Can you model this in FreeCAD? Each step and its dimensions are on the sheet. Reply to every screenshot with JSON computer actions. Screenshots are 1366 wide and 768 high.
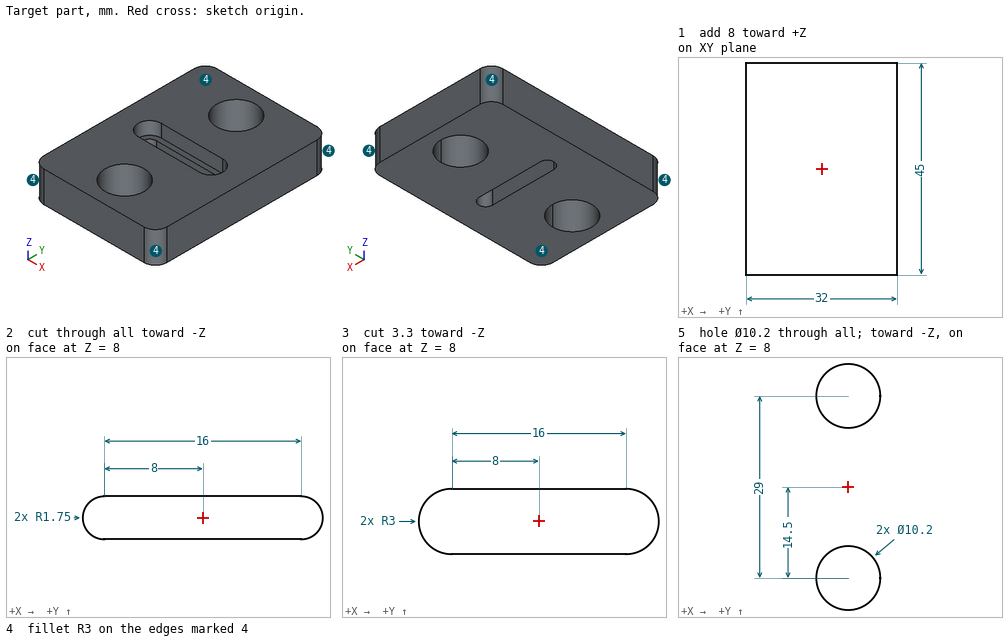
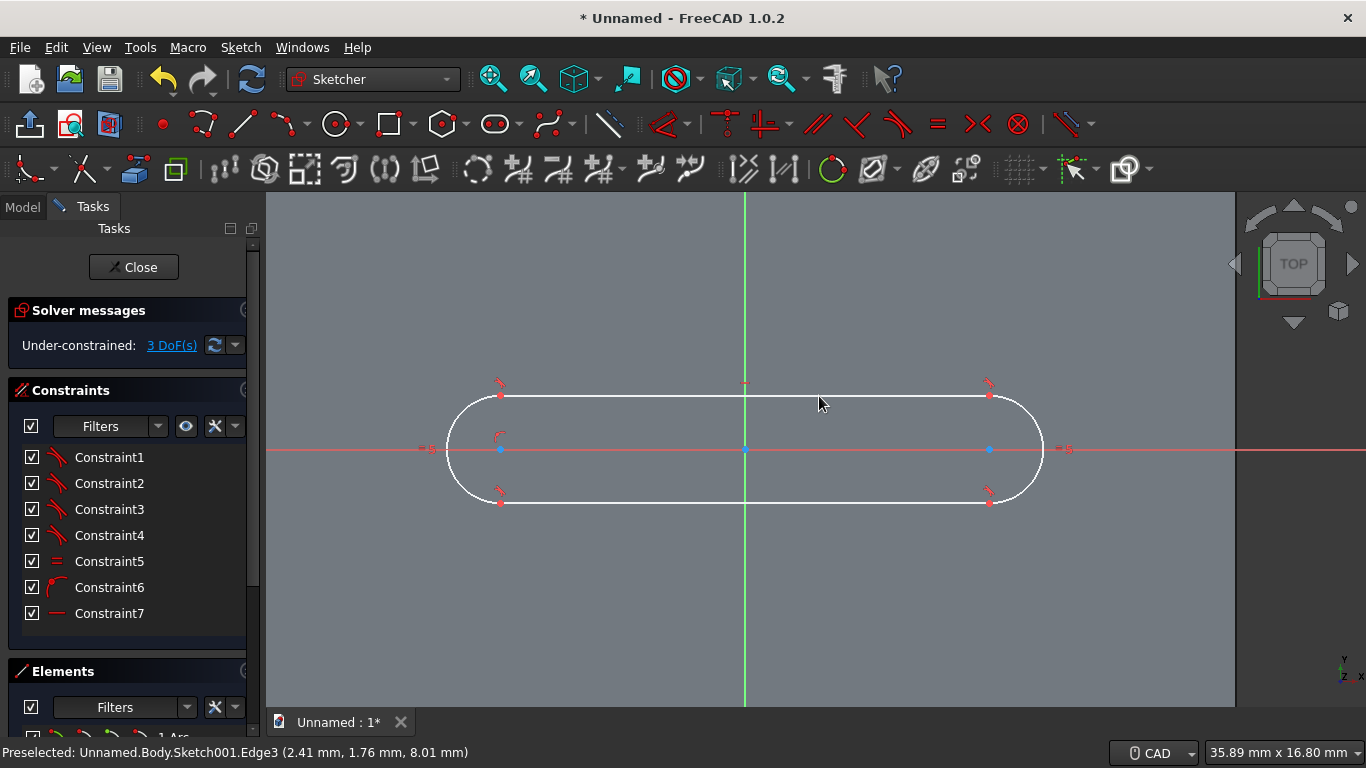
{"action": "key", "text": "d"}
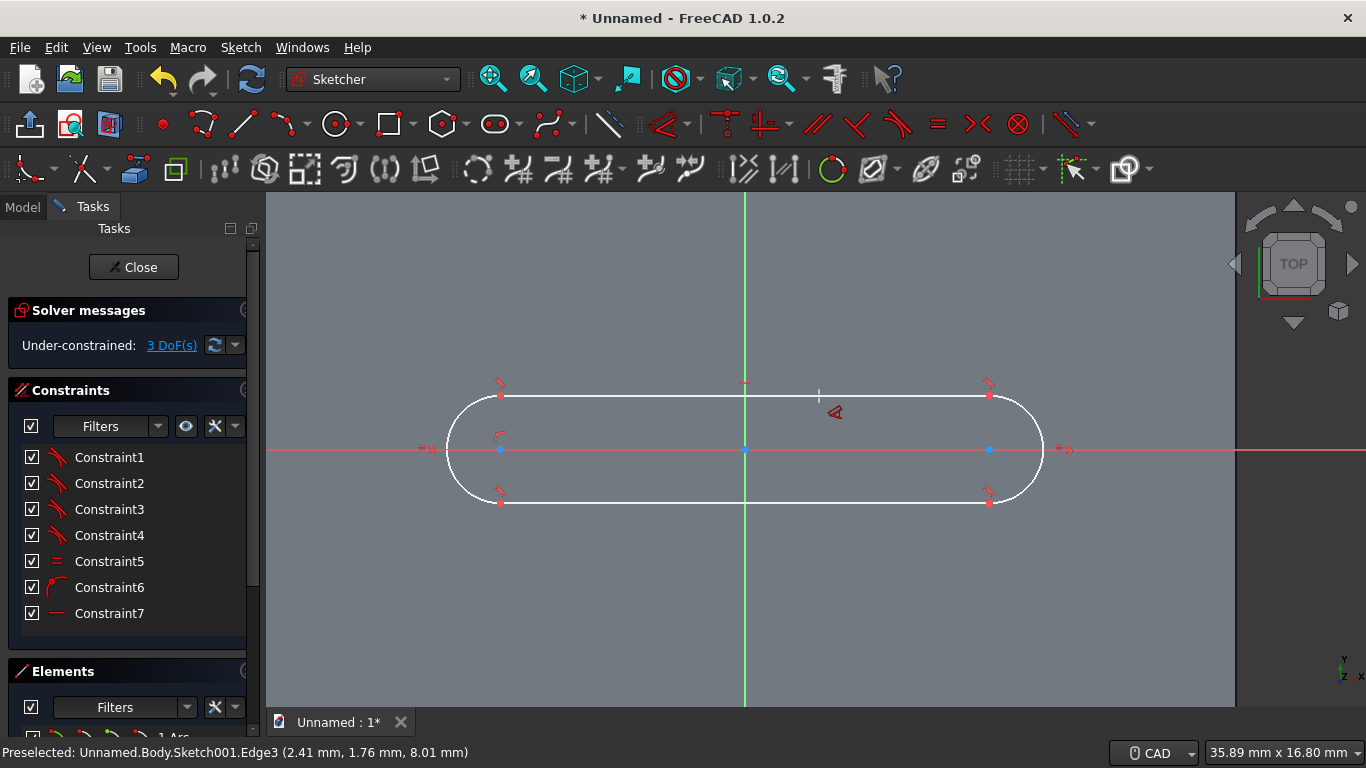
{"action": "left_click", "coordinate": [457, 418]}
{"action": "left_click", "coordinate": [431, 399]}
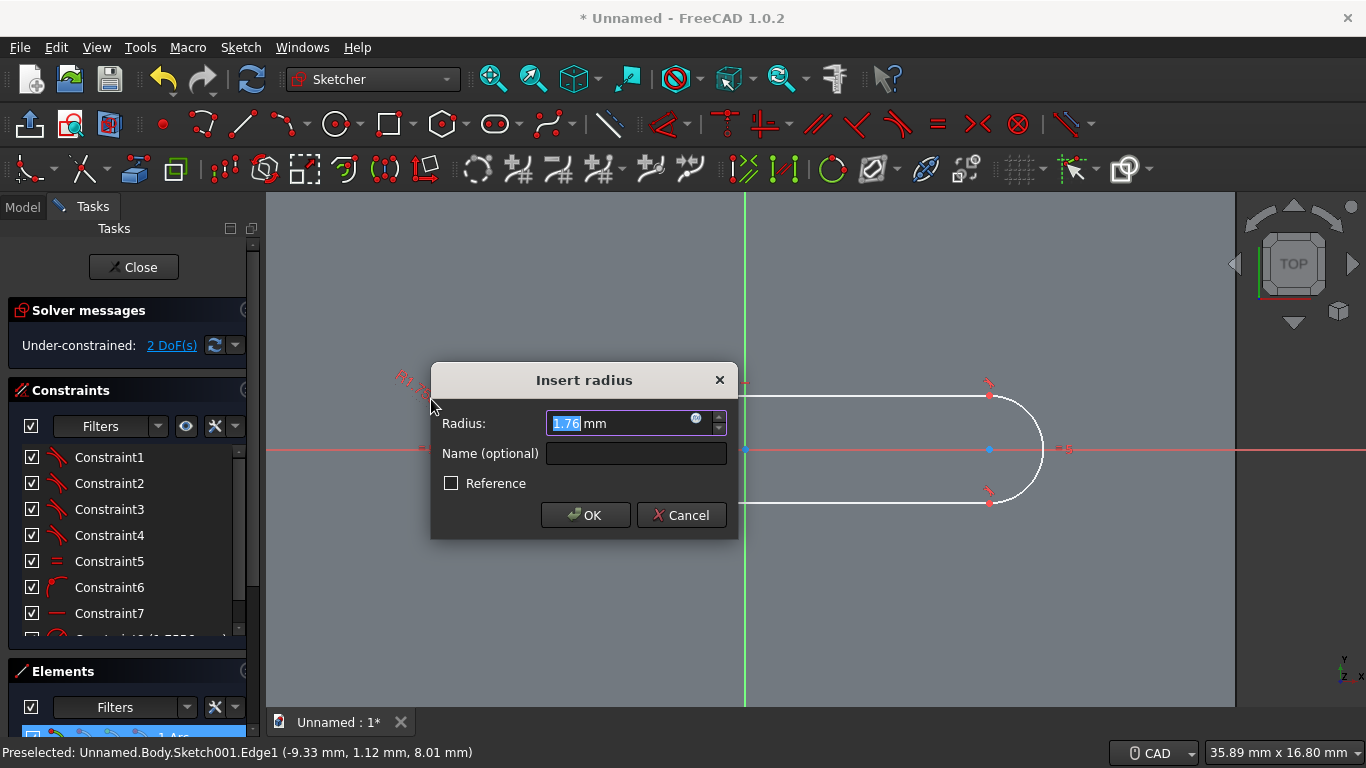
{"action": "type", "text": "1.75"}
{"action": "key", "text": "Return"}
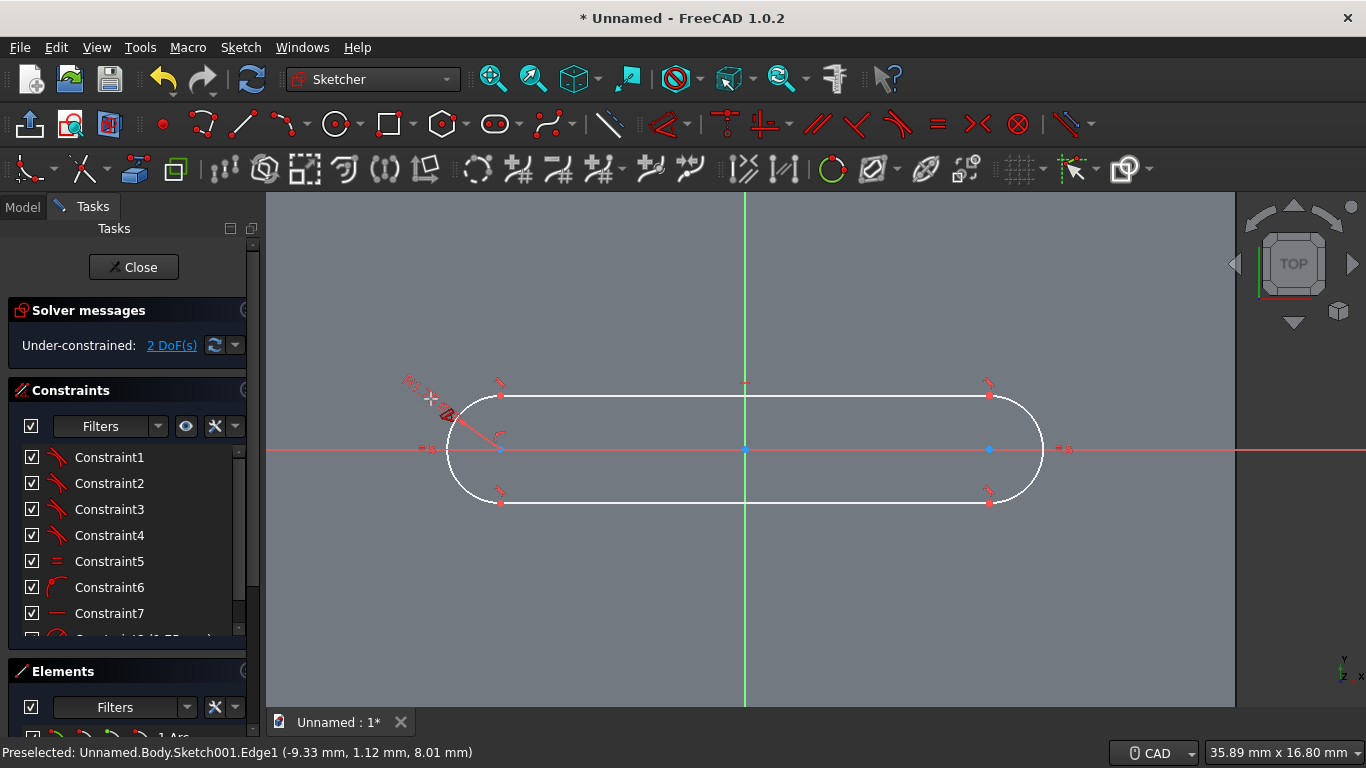
{"action": "left_click", "coordinate": [647, 396]}
{"action": "left_click", "coordinate": [633, 362]}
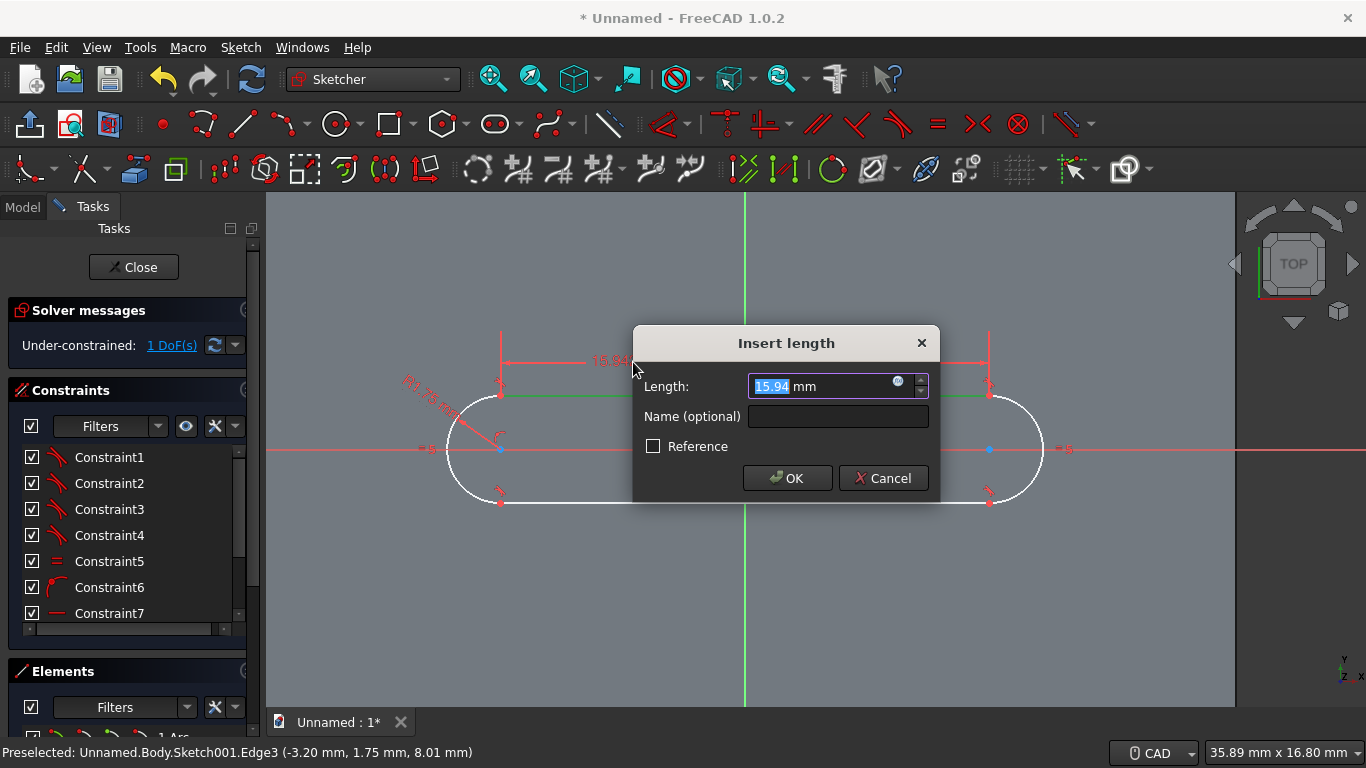
{"action": "type", "text": "16"}
{"action": "key", "text": "Return"}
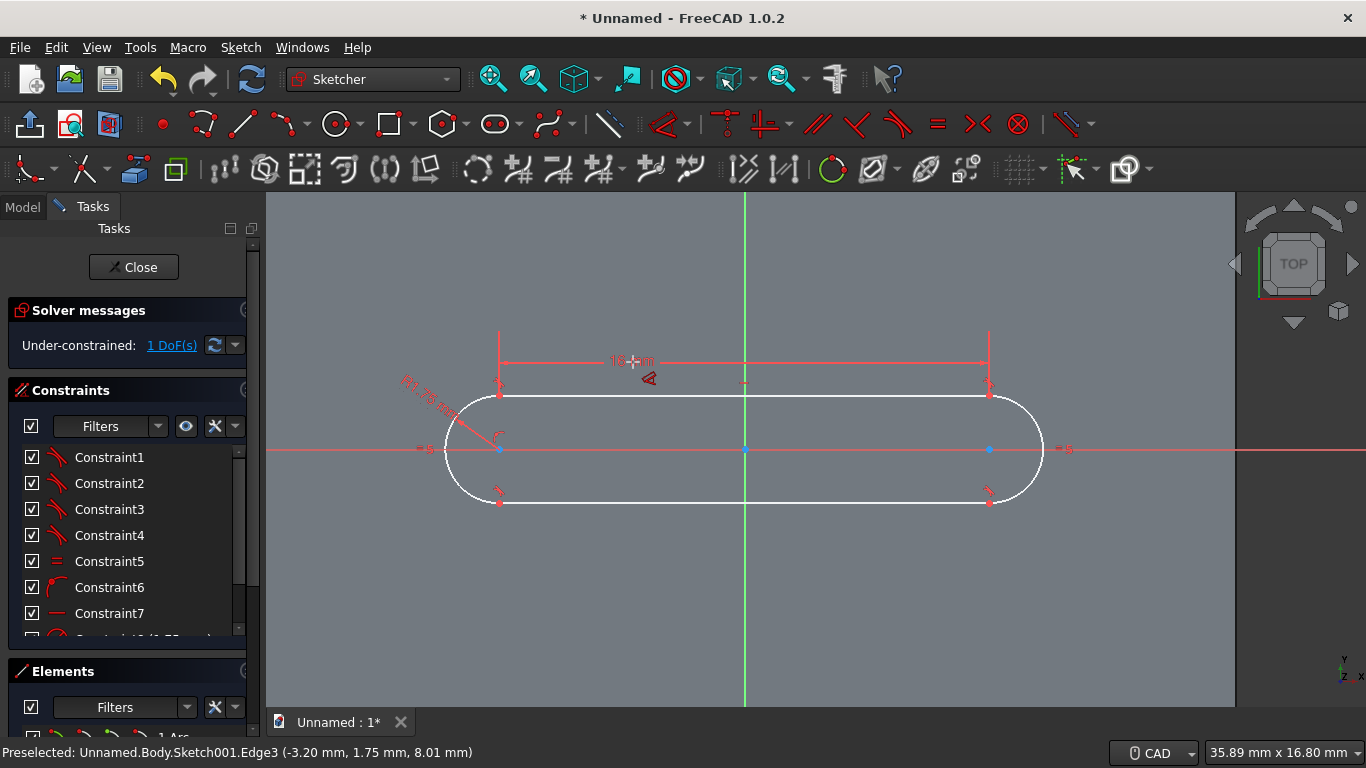
{"action": "left_click", "coordinate": [499, 396]}
{"action": "left_click", "coordinate": [536, 362]}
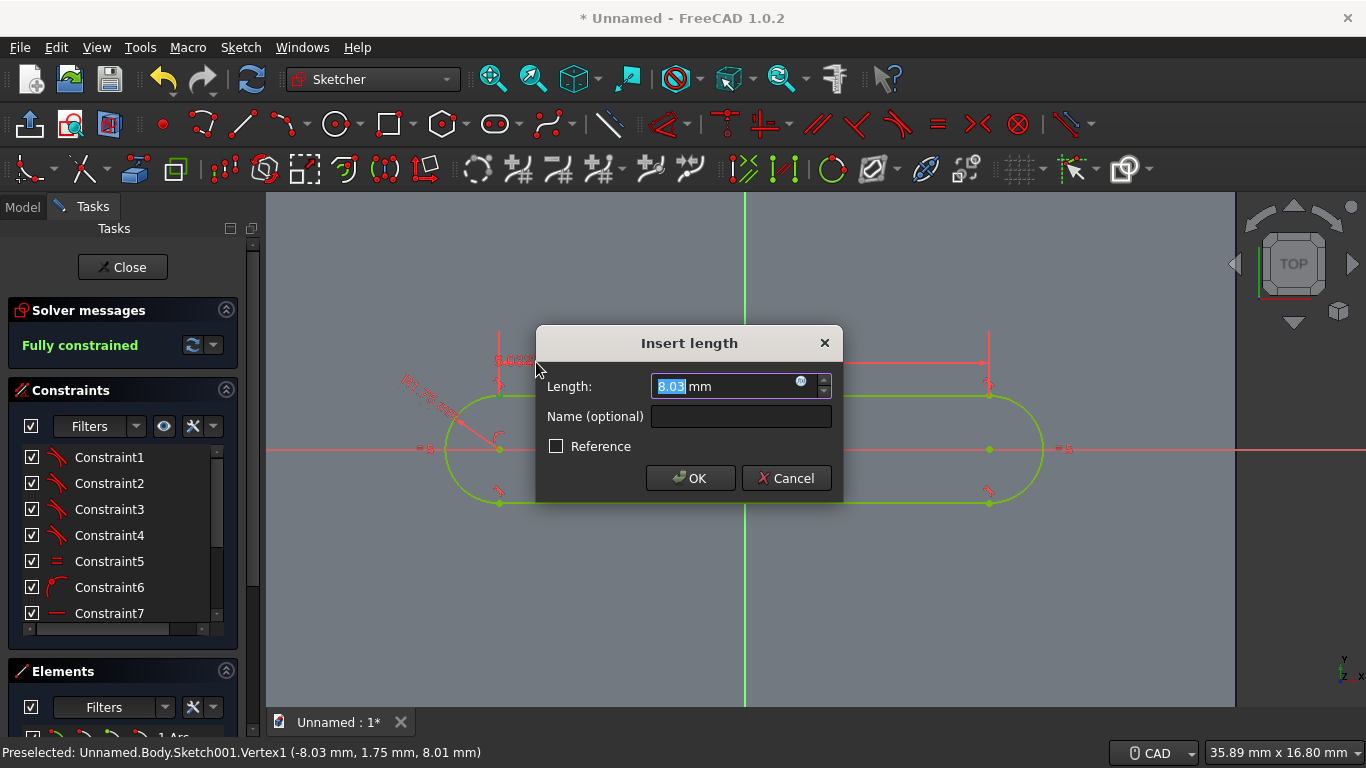
{"action": "type", "text": "8"}
{"action": "key", "text": "Return"}
{"action": "key", "text": "Escape"}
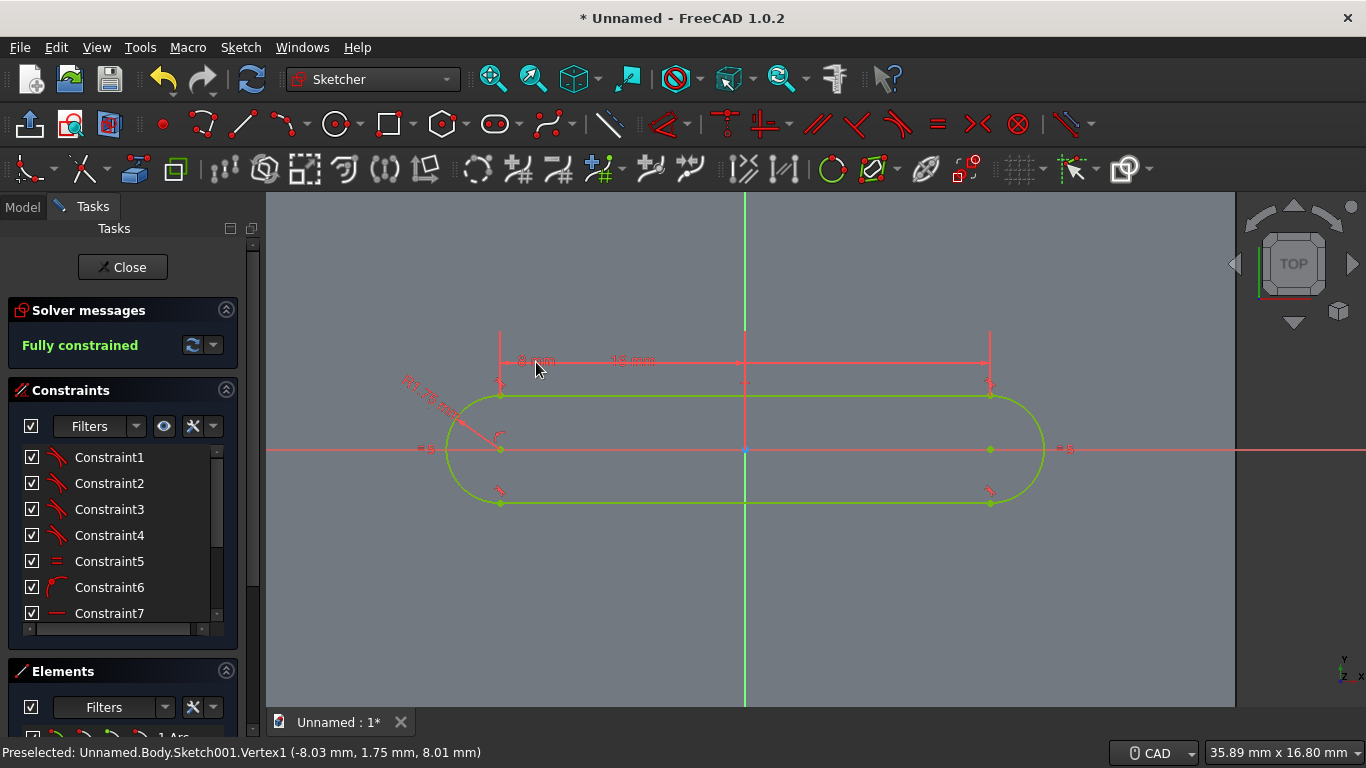
{"action": "left_click", "coordinate": [123, 267]}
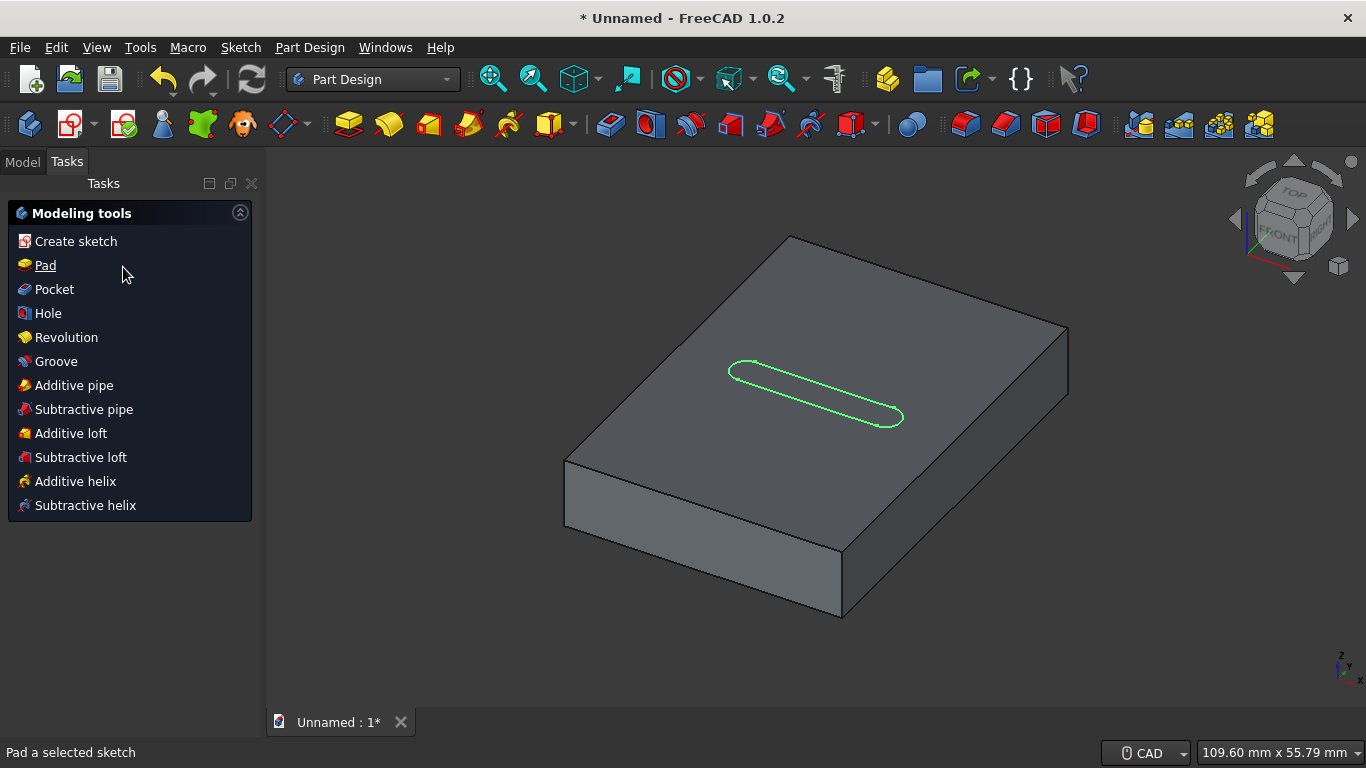
{"action": "left_click", "coordinate": [612, 124]}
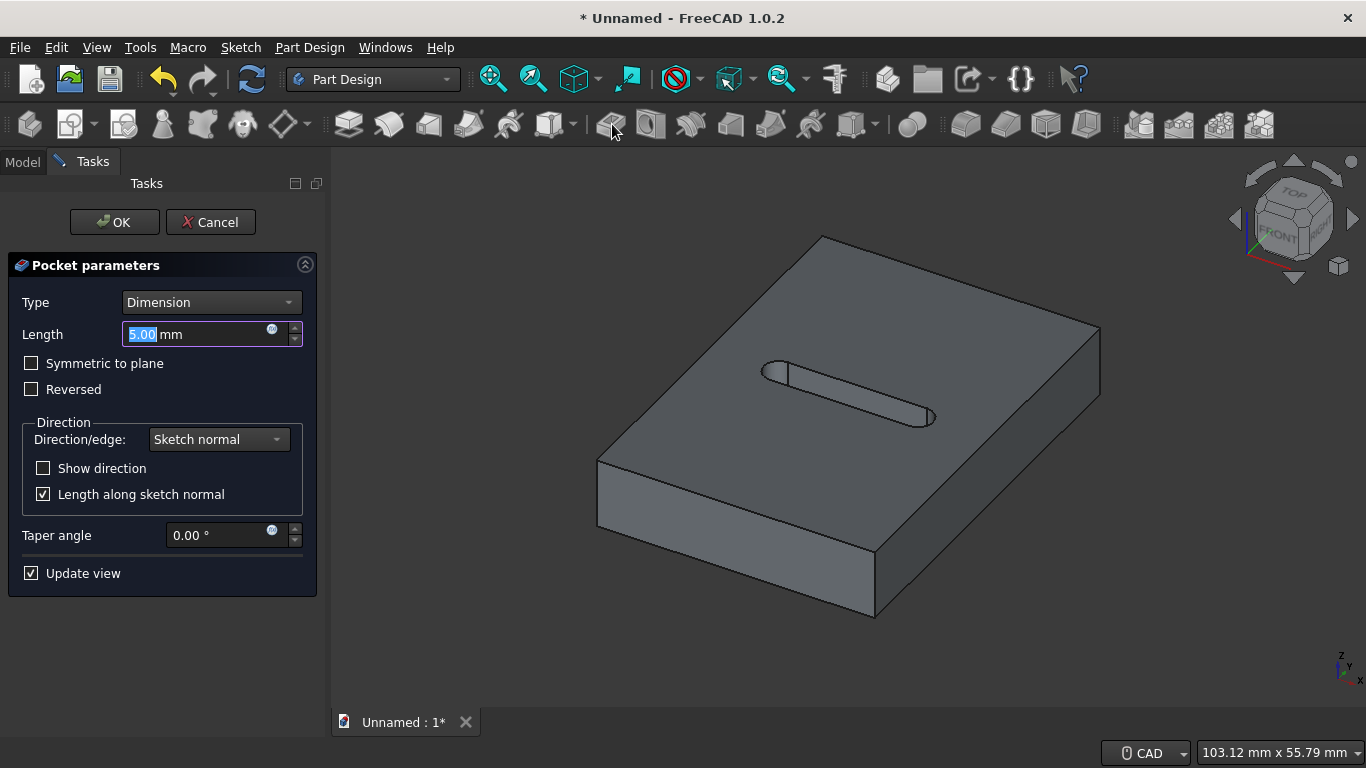
{"action": "left_click", "coordinate": [212, 302]}